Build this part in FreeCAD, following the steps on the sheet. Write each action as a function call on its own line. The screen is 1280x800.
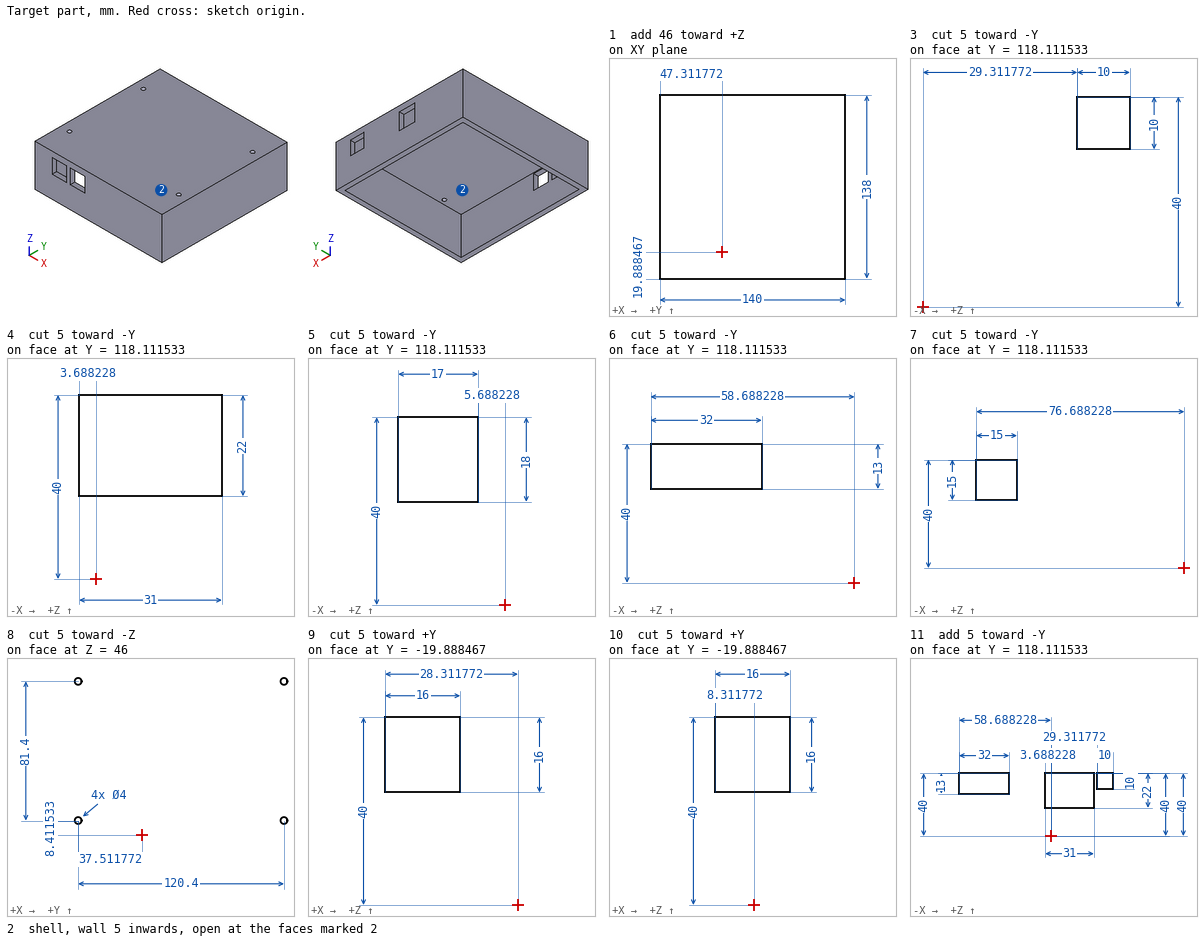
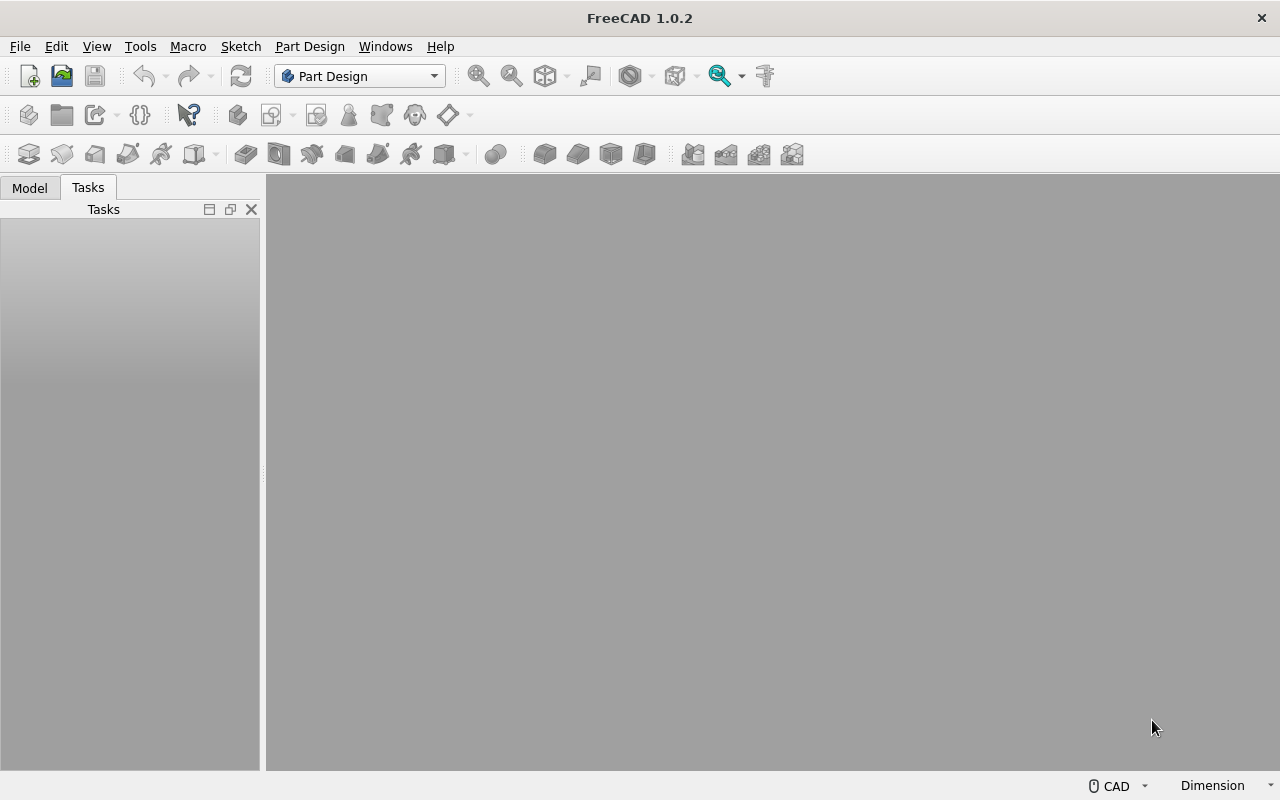
key(ctrl+n)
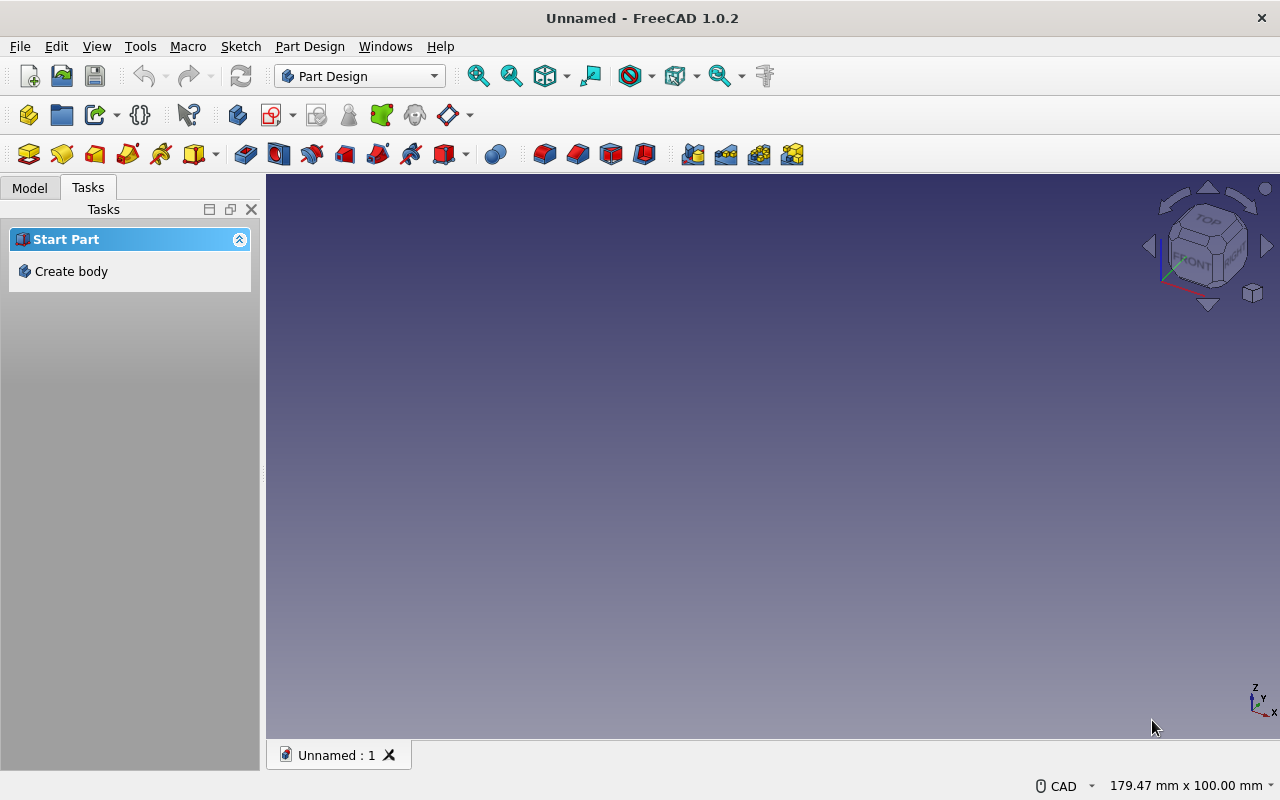
click(270, 116)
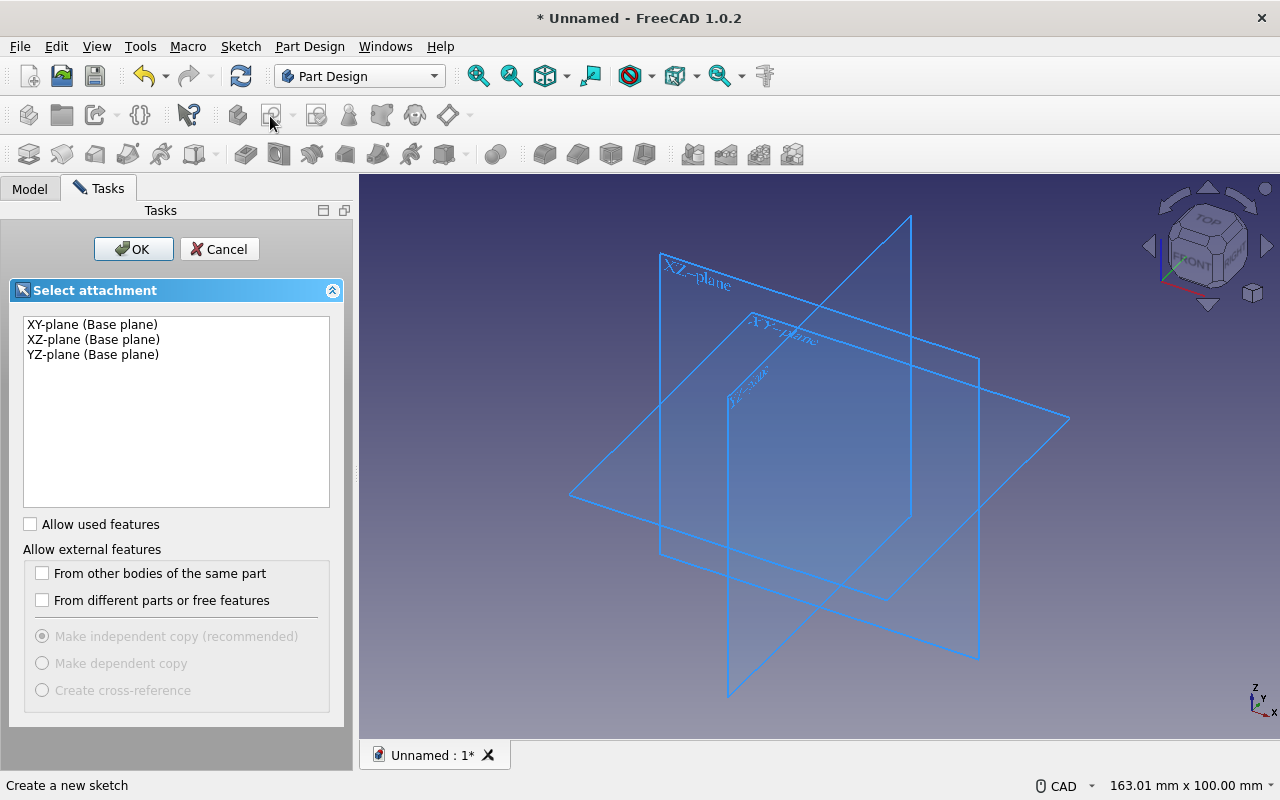
click(84, 324)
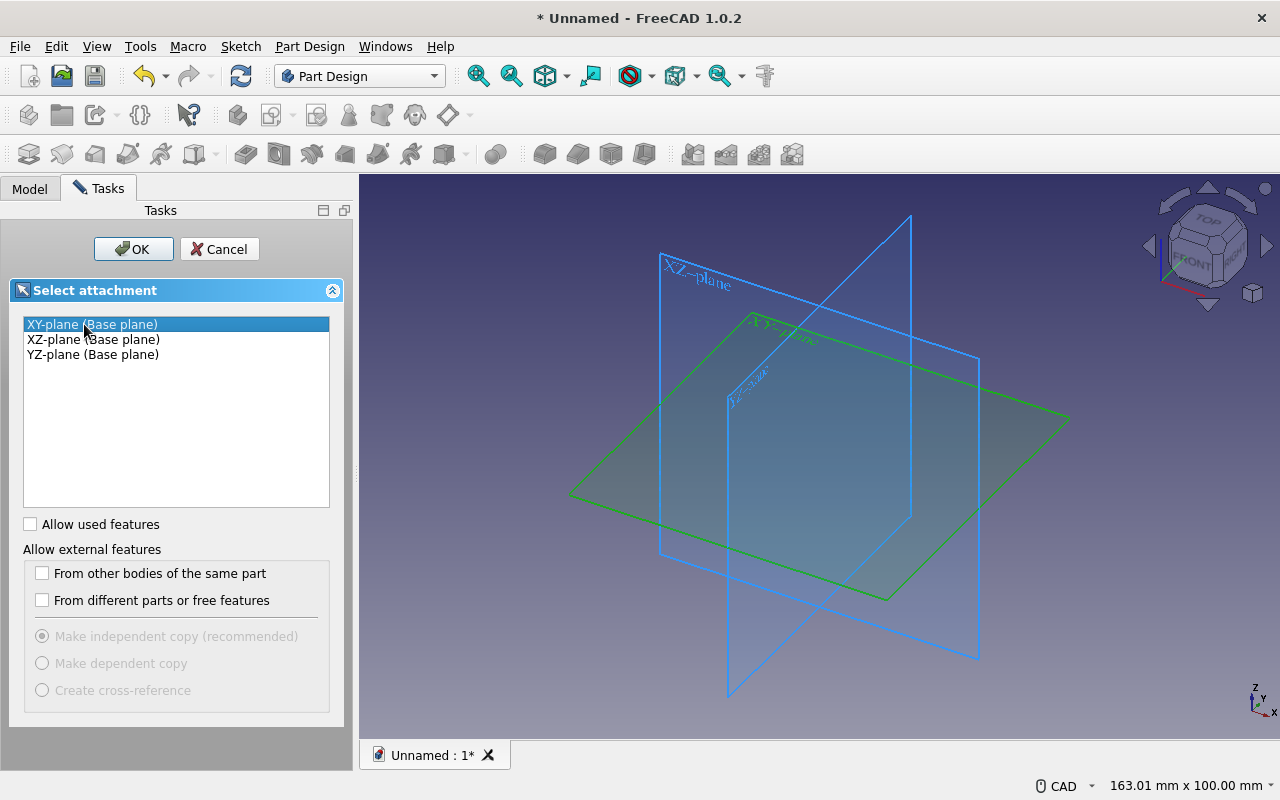
click(134, 249)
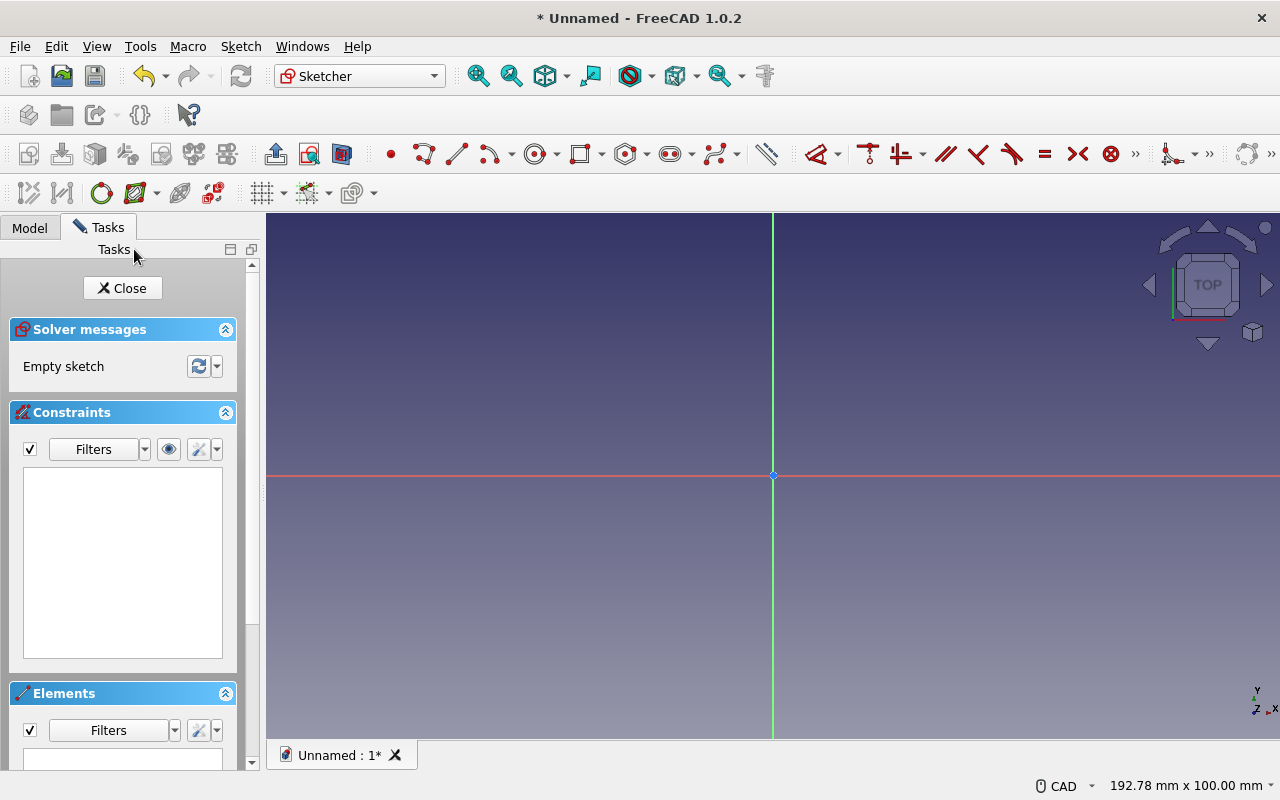
scroll(551, 687, down, 4)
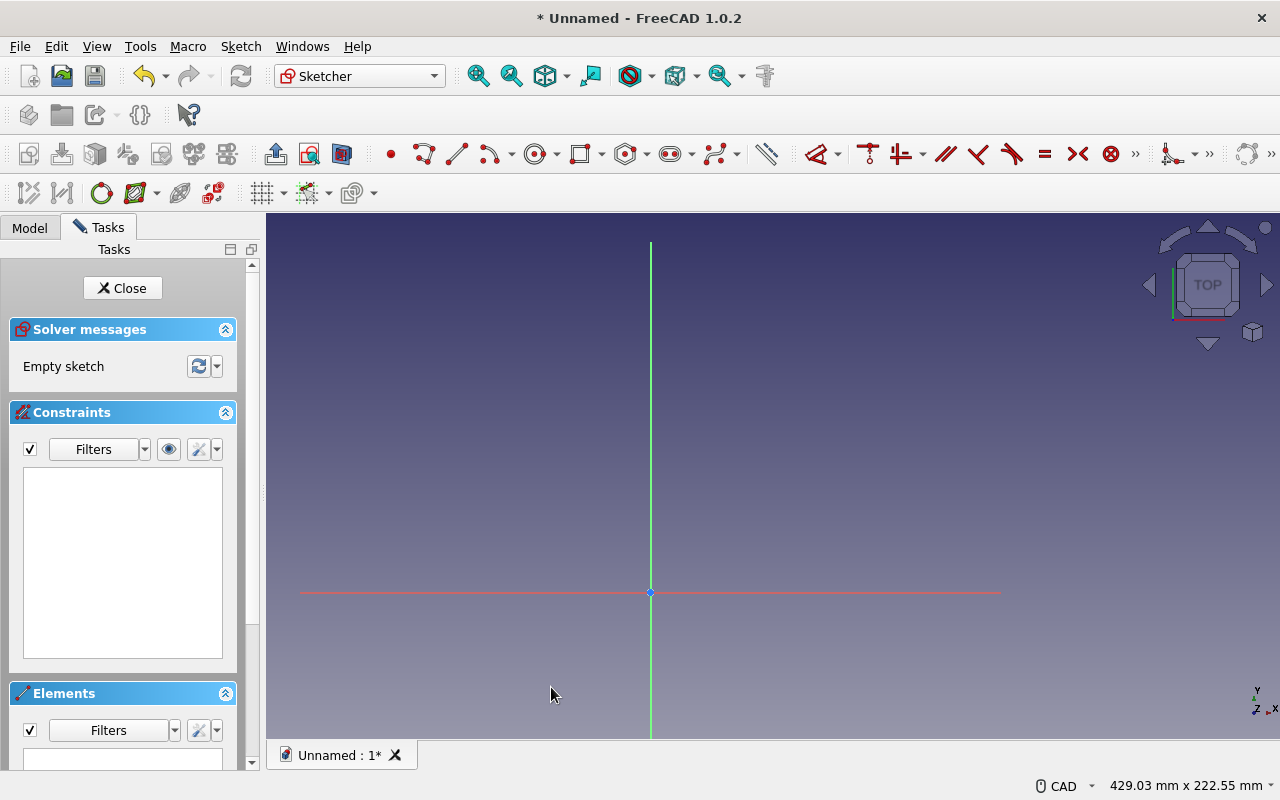
key(g)
key(r)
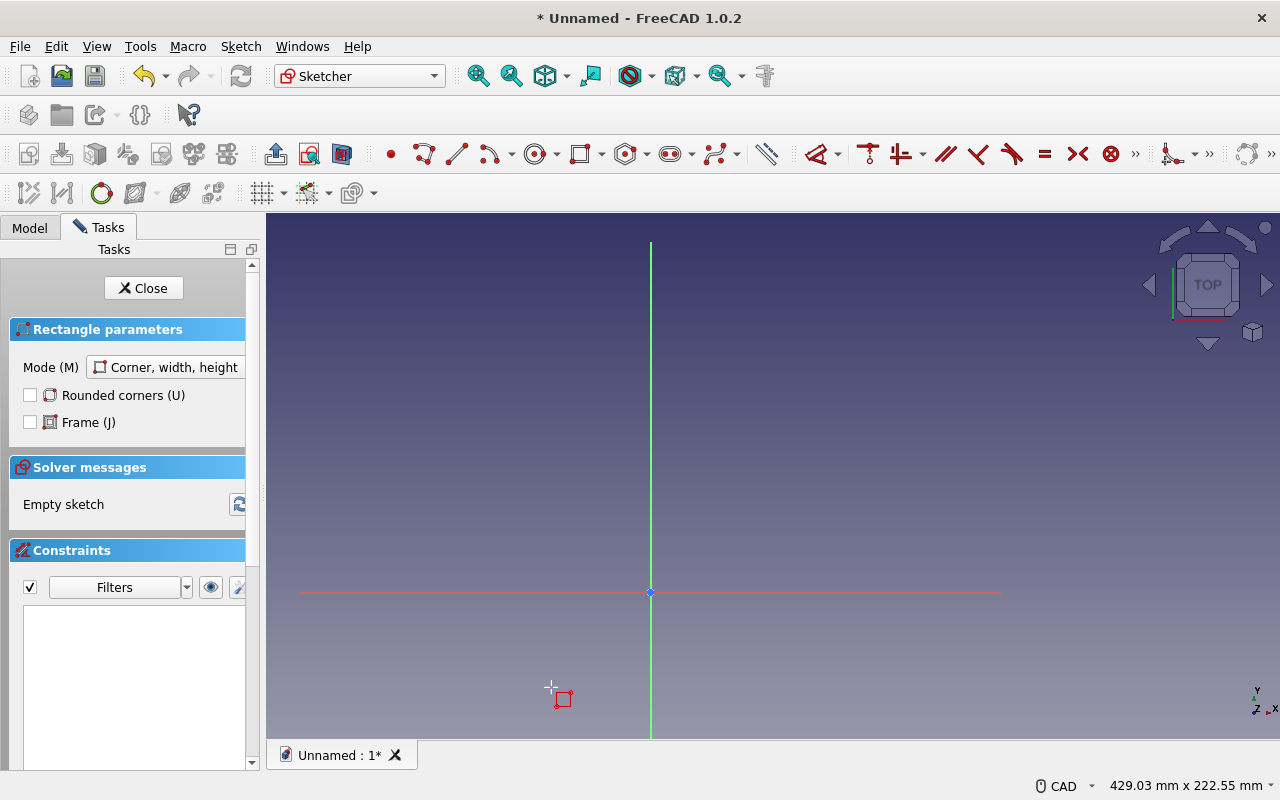
click(539, 314)
move(870, 640)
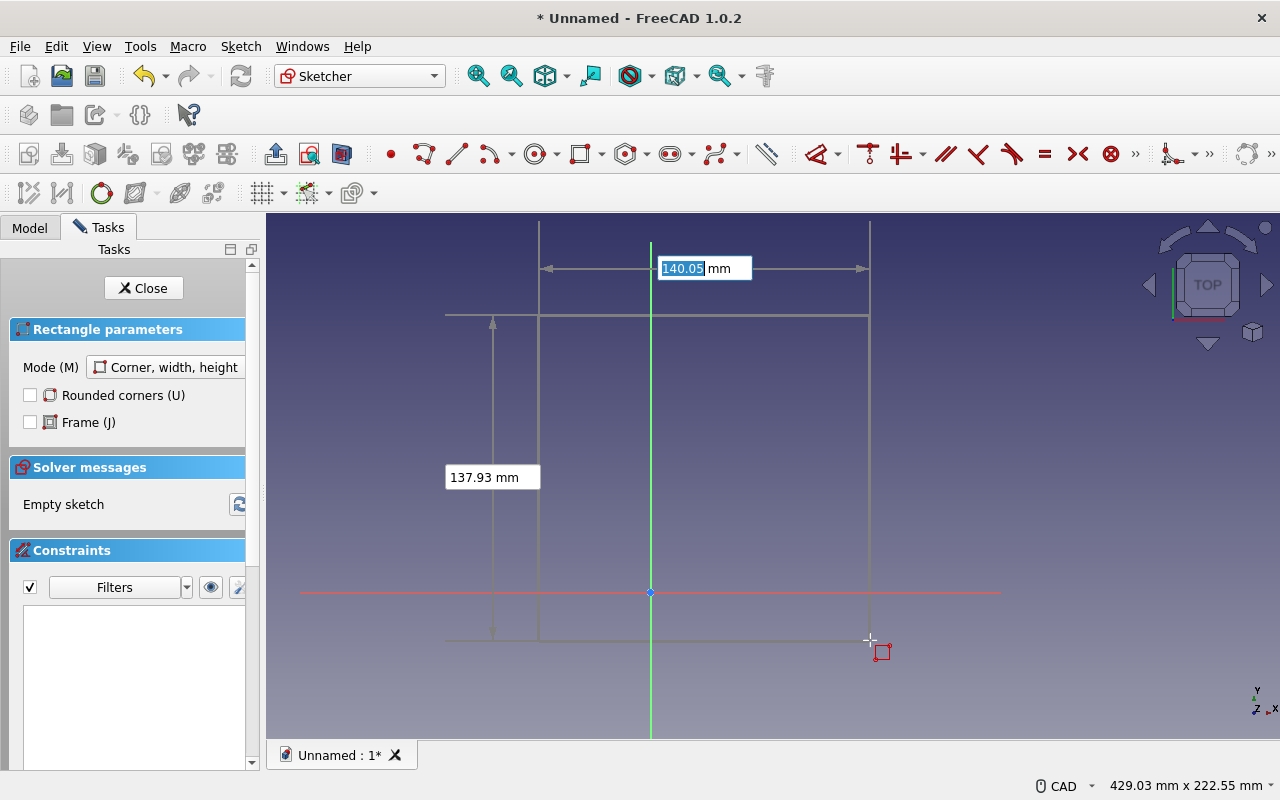
text(140)
key(Tab)
text(138)
key(Return)
key(Escape)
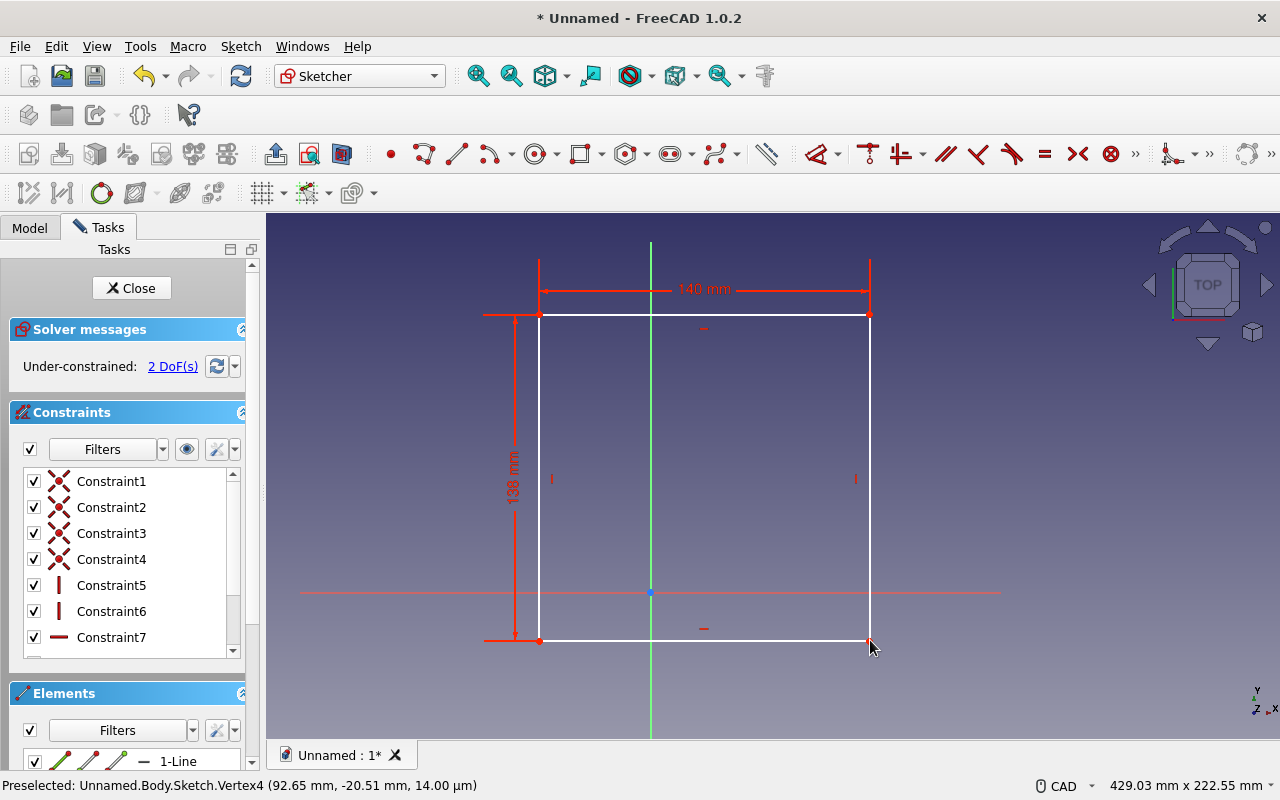
key(d)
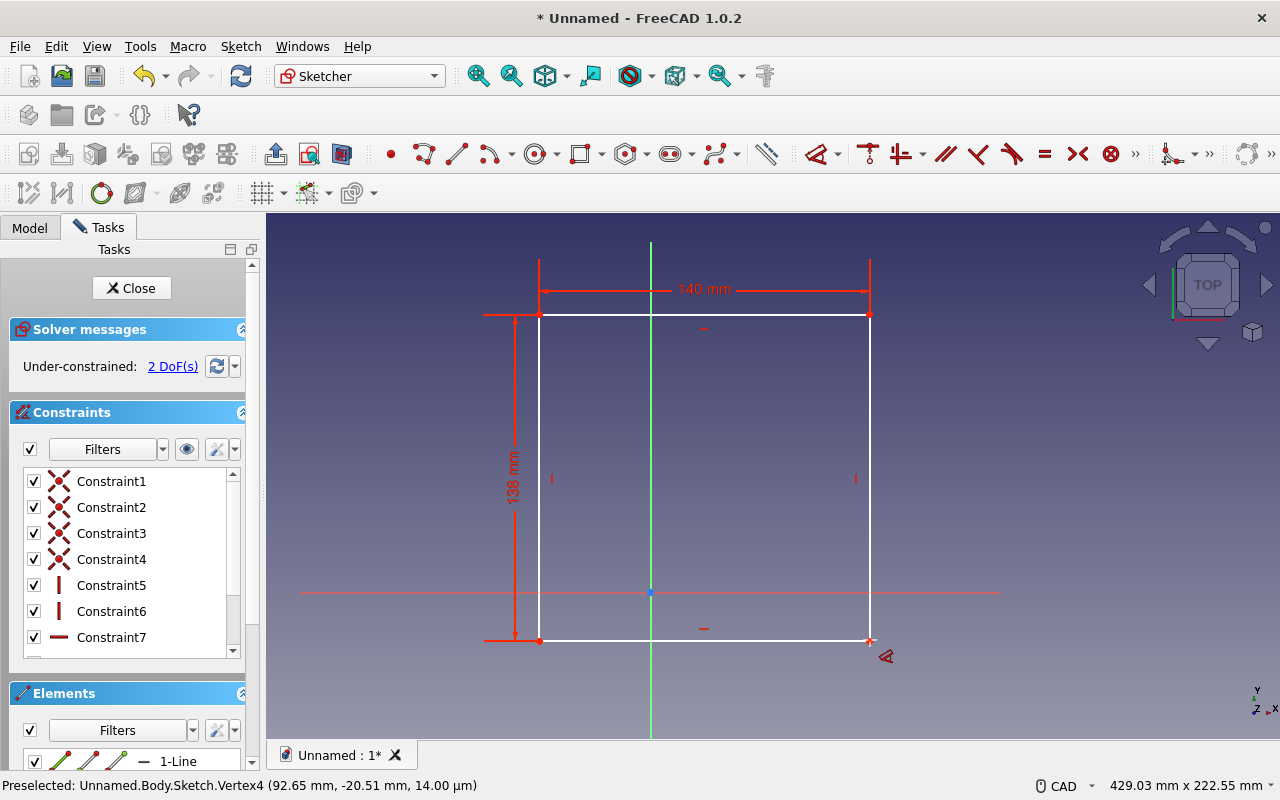
click(539, 315)
click(595, 281)